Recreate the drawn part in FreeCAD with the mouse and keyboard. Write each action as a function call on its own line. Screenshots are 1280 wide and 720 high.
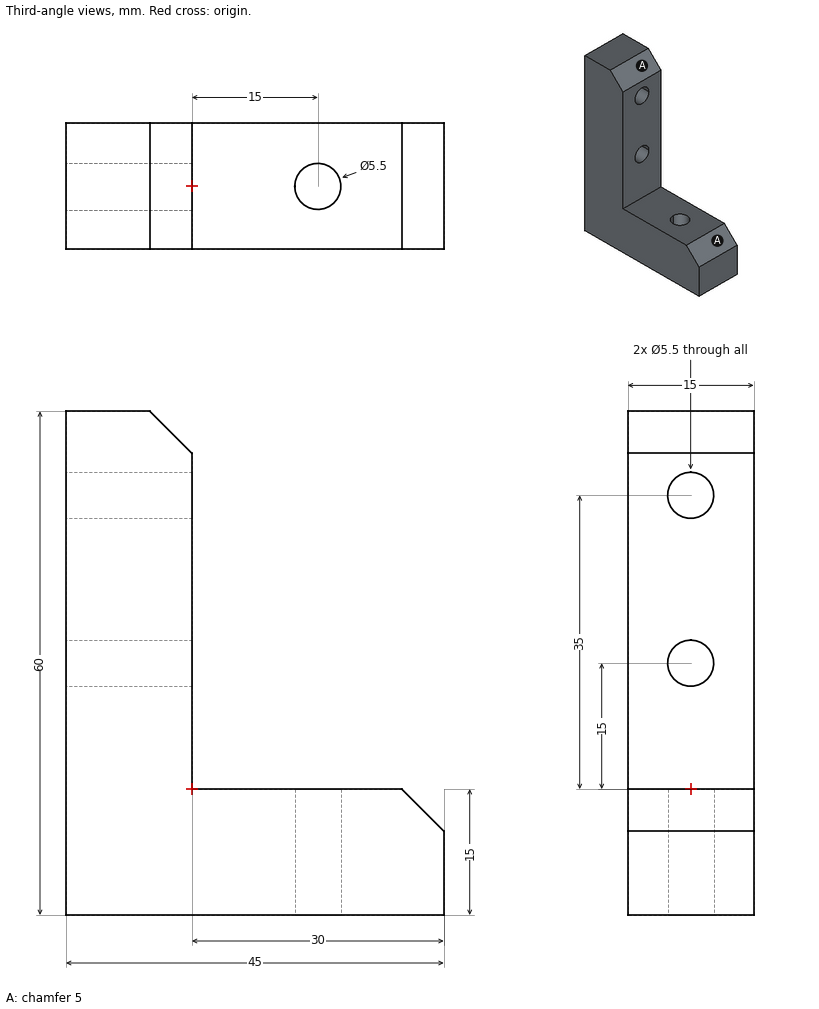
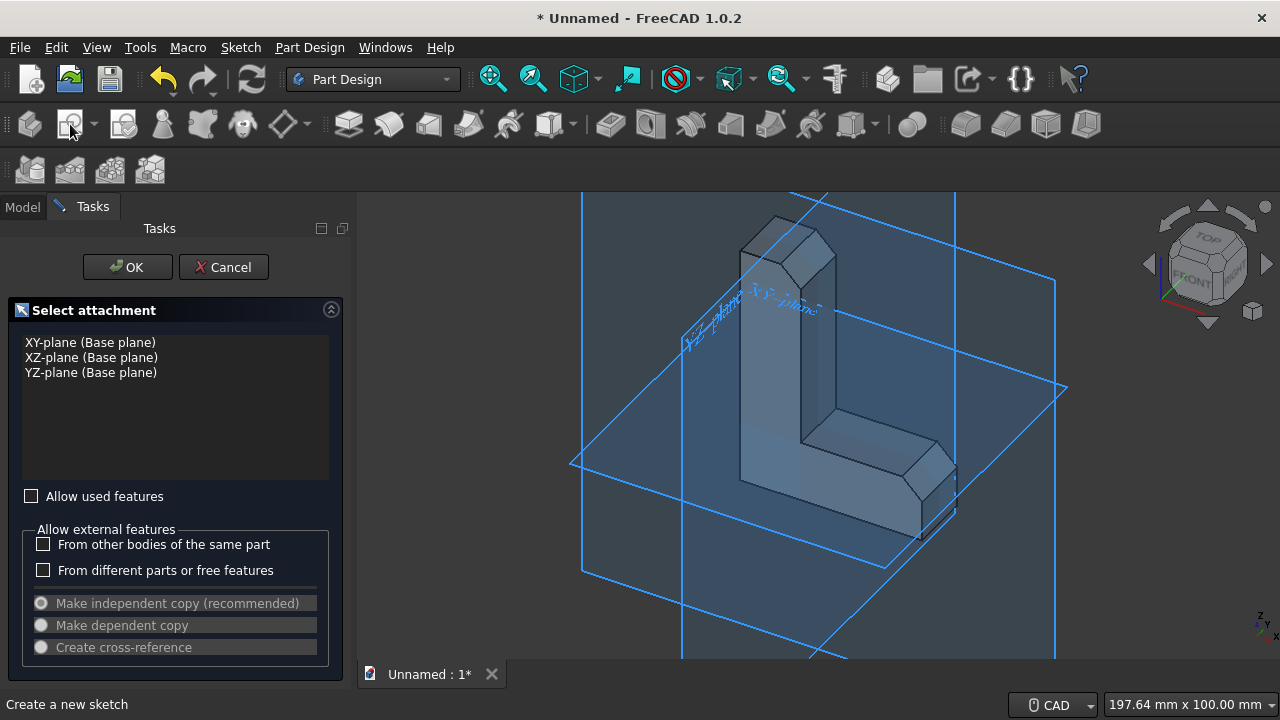
click(82, 372)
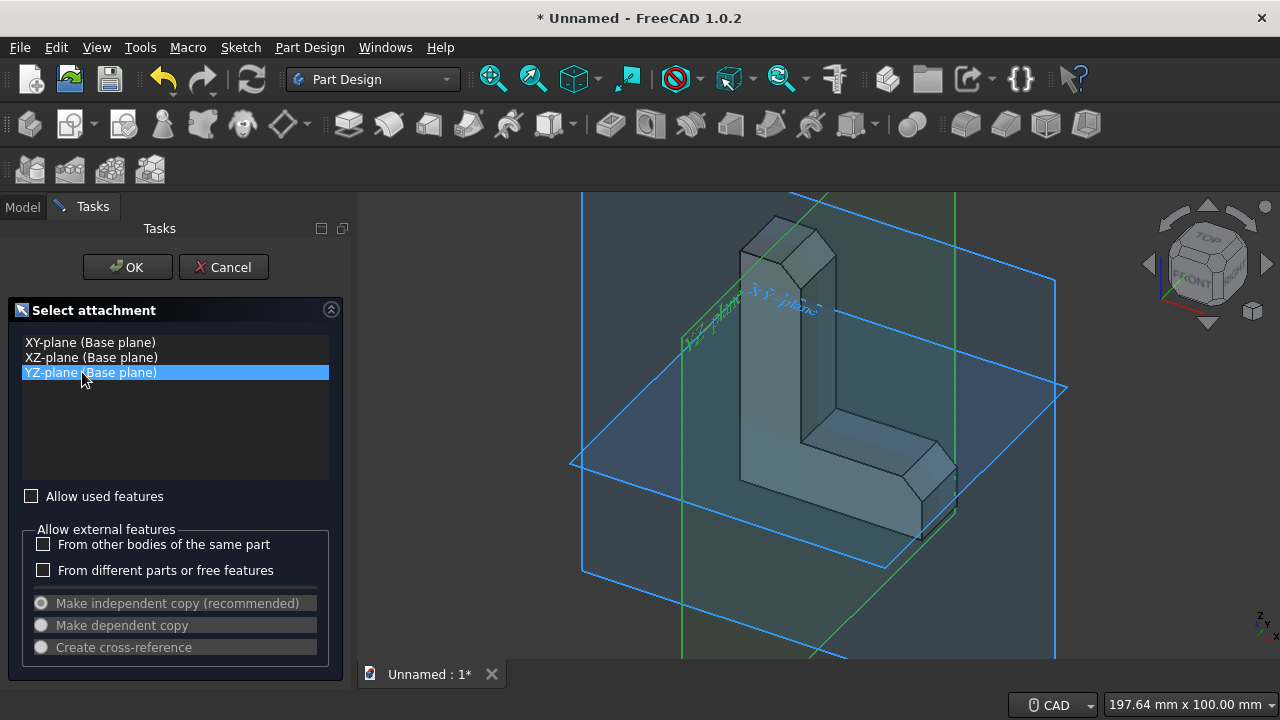
click(128, 267)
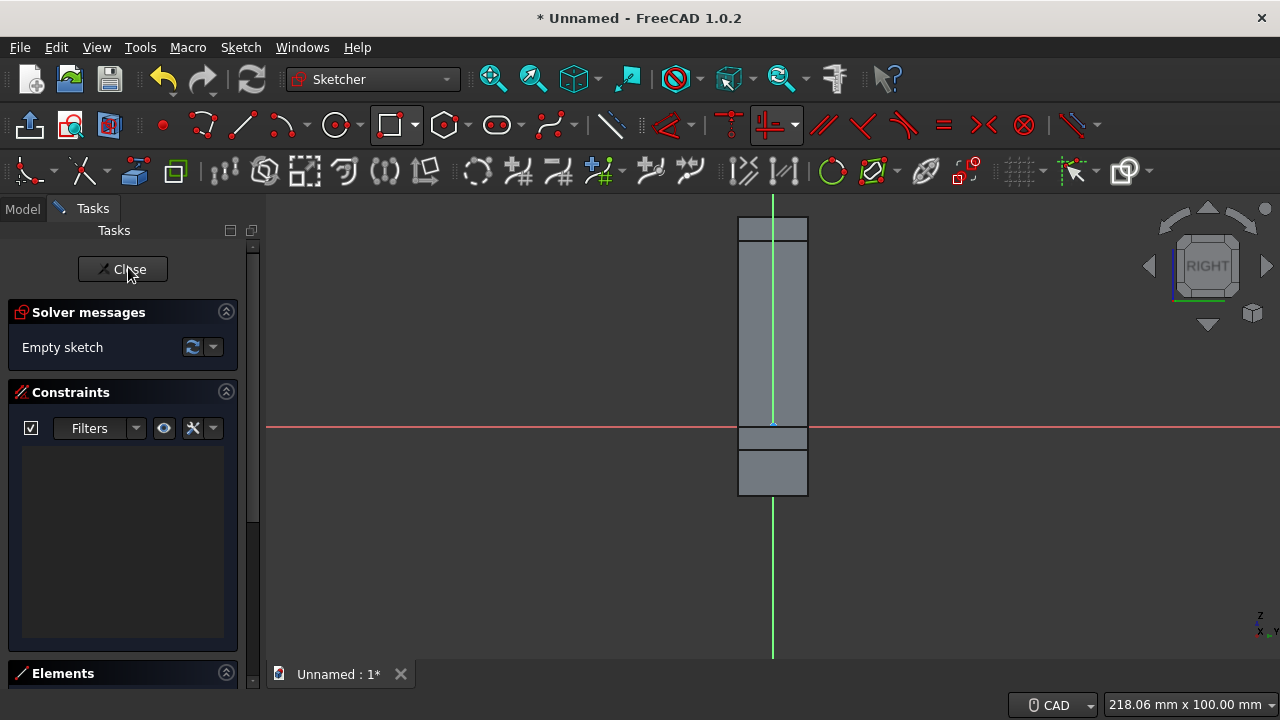
key(q)
key(s)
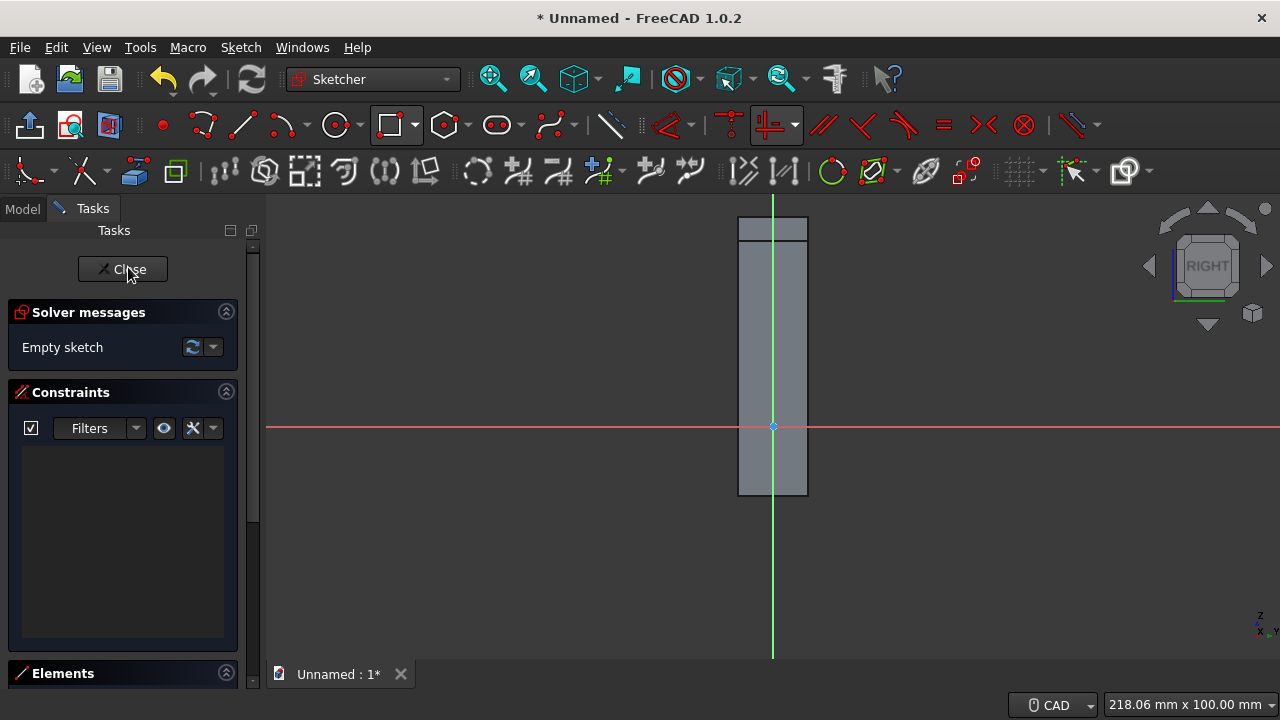
scroll(912, 222, up, 2)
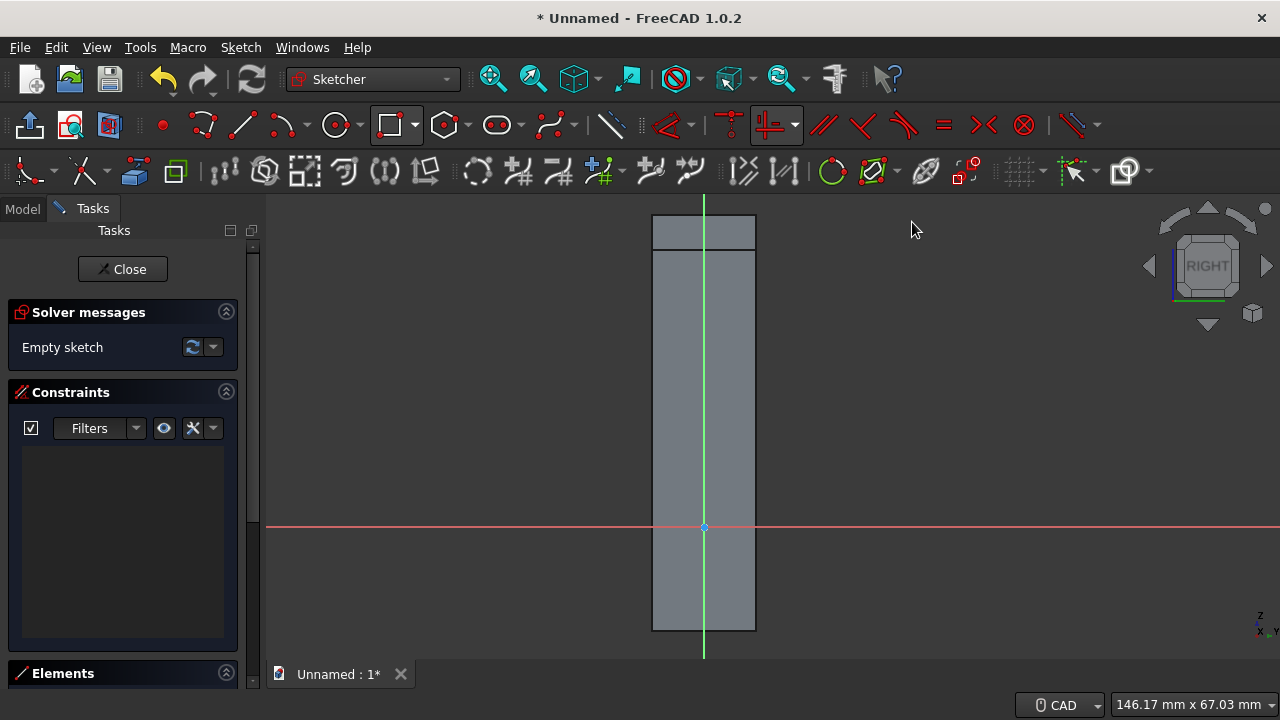
key(g)
key(c)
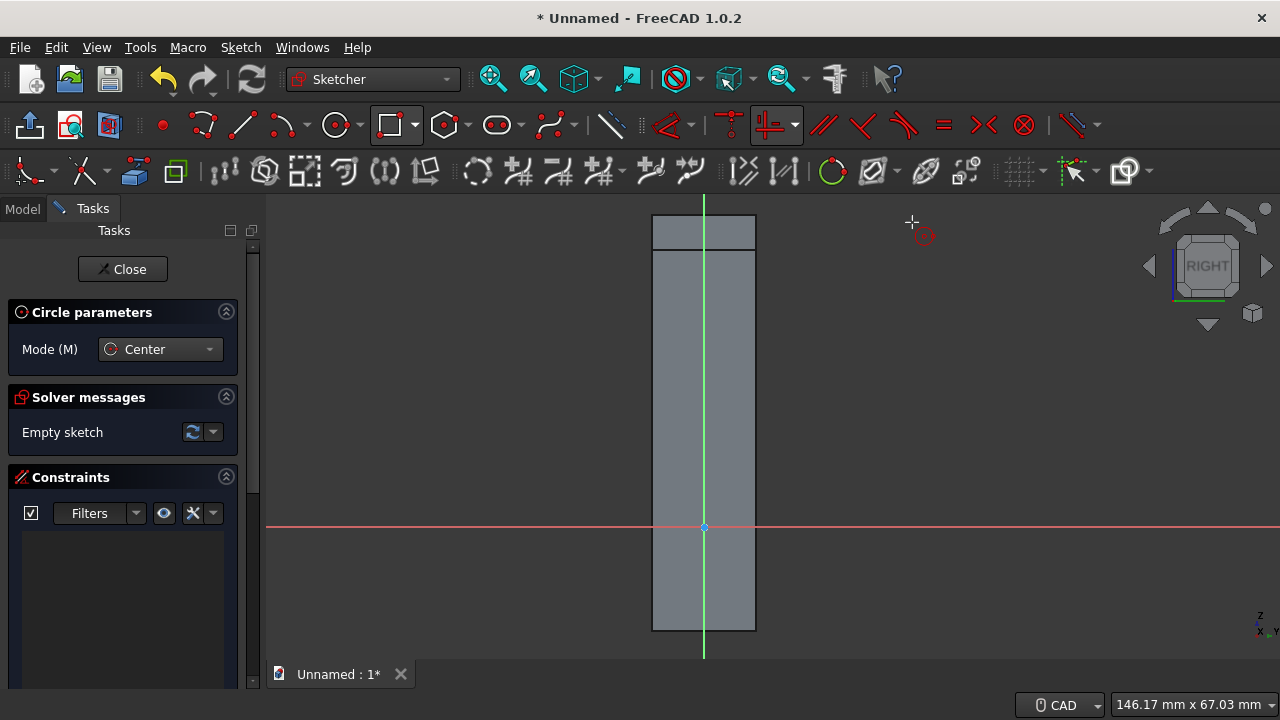
click(704, 284)
move(722, 278)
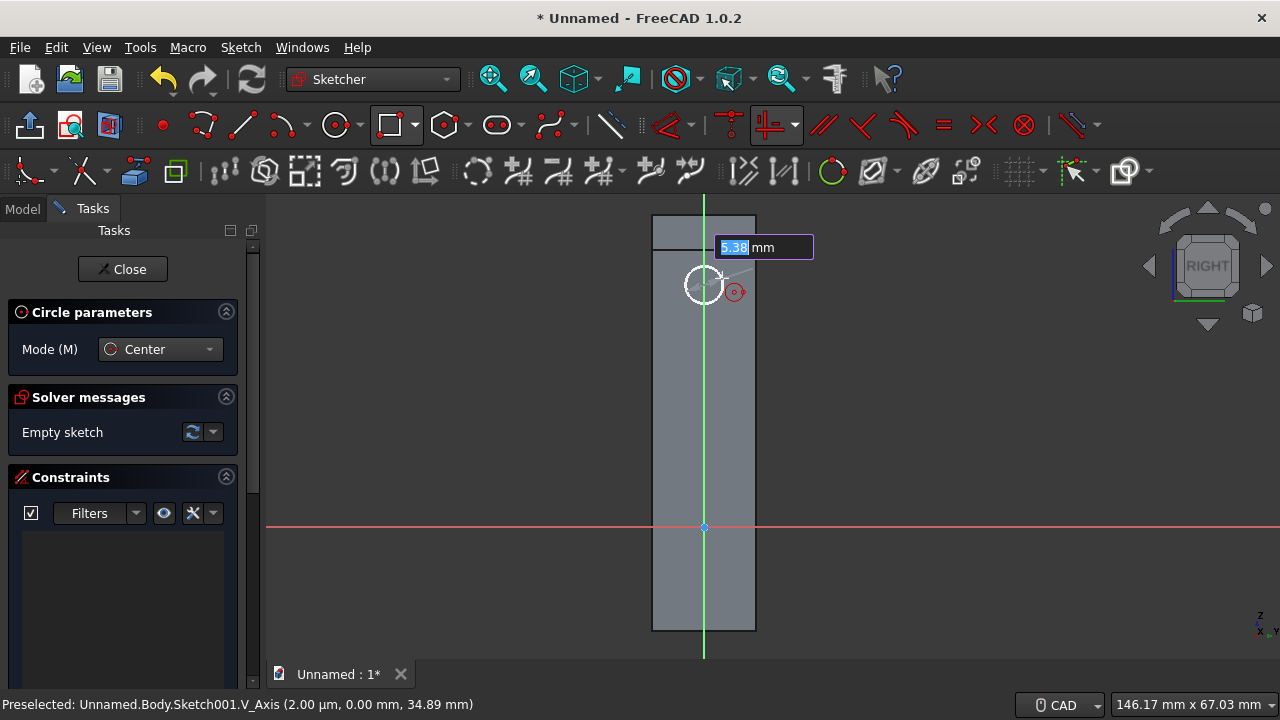
text(5.5)
key(Return)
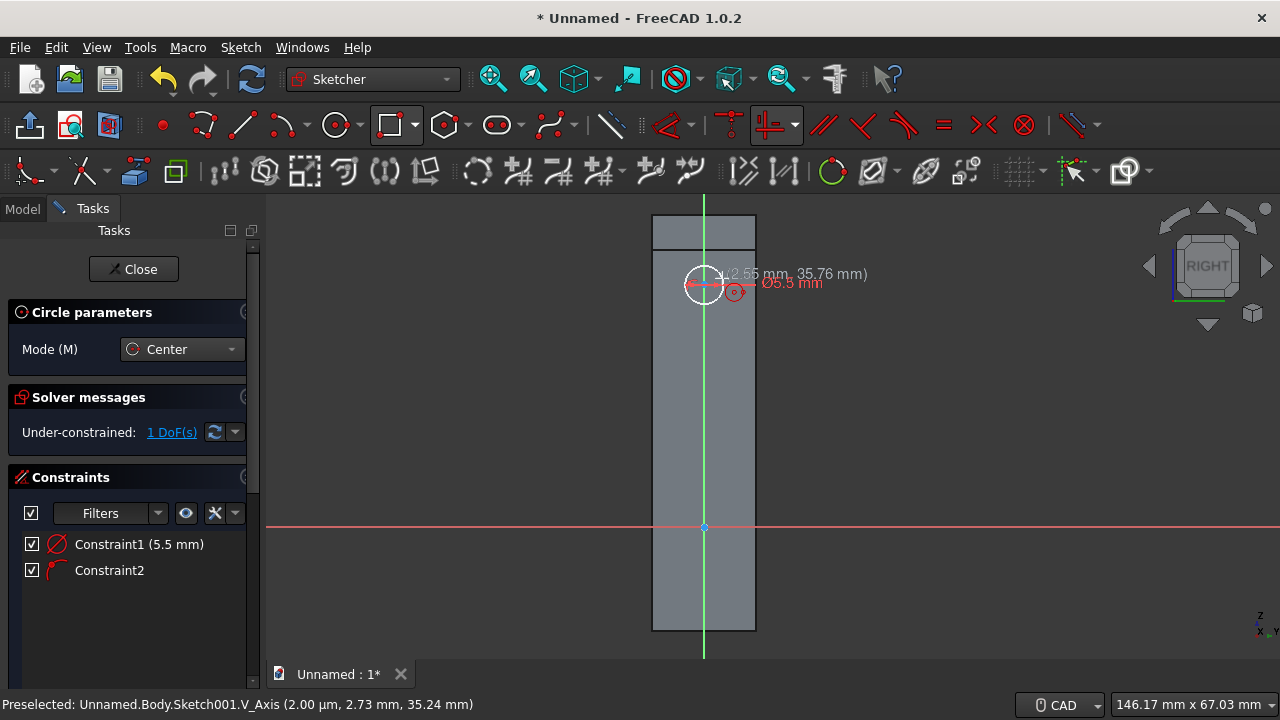
click(704, 423)
move(722, 416)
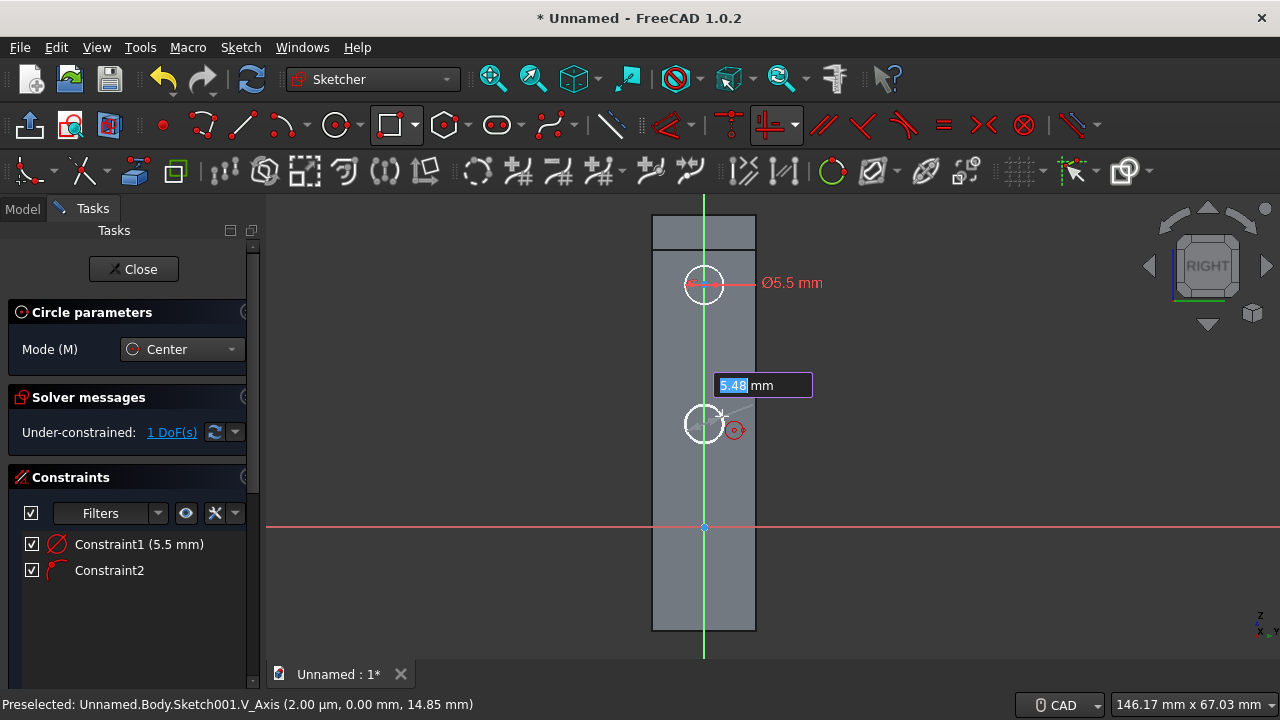
text(5.5)
key(Return)
key(Escape)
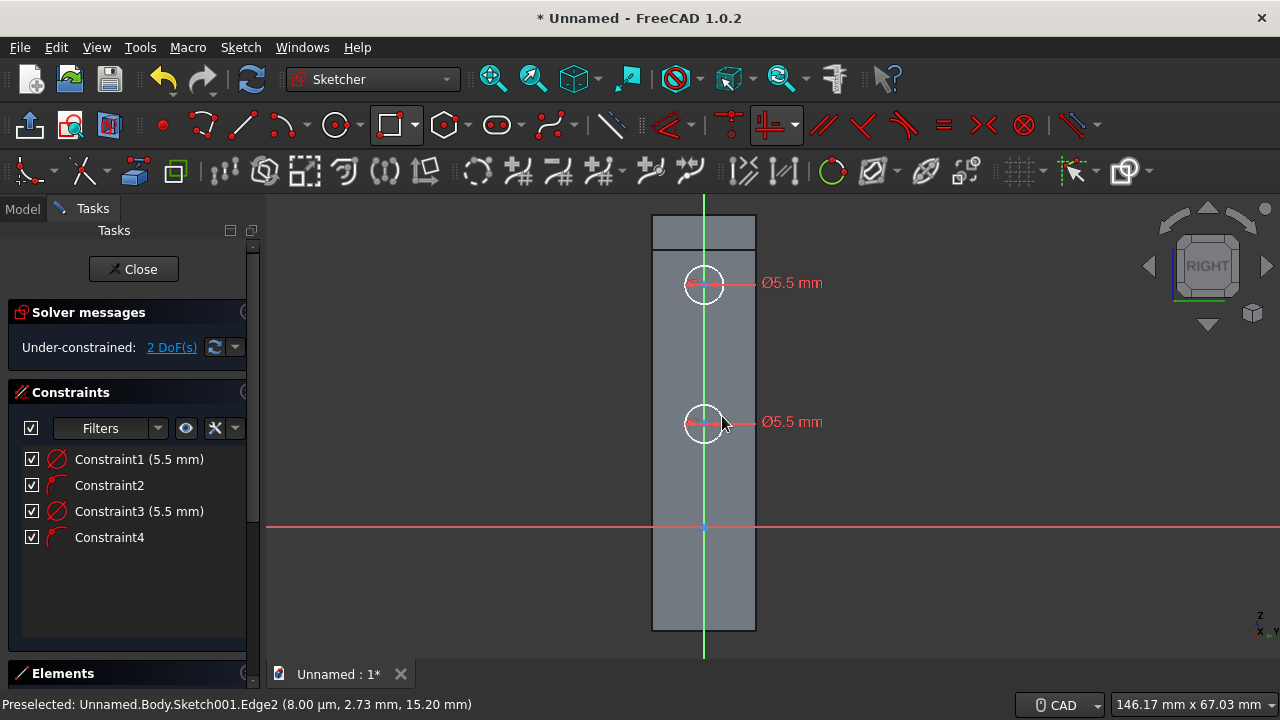
key(d)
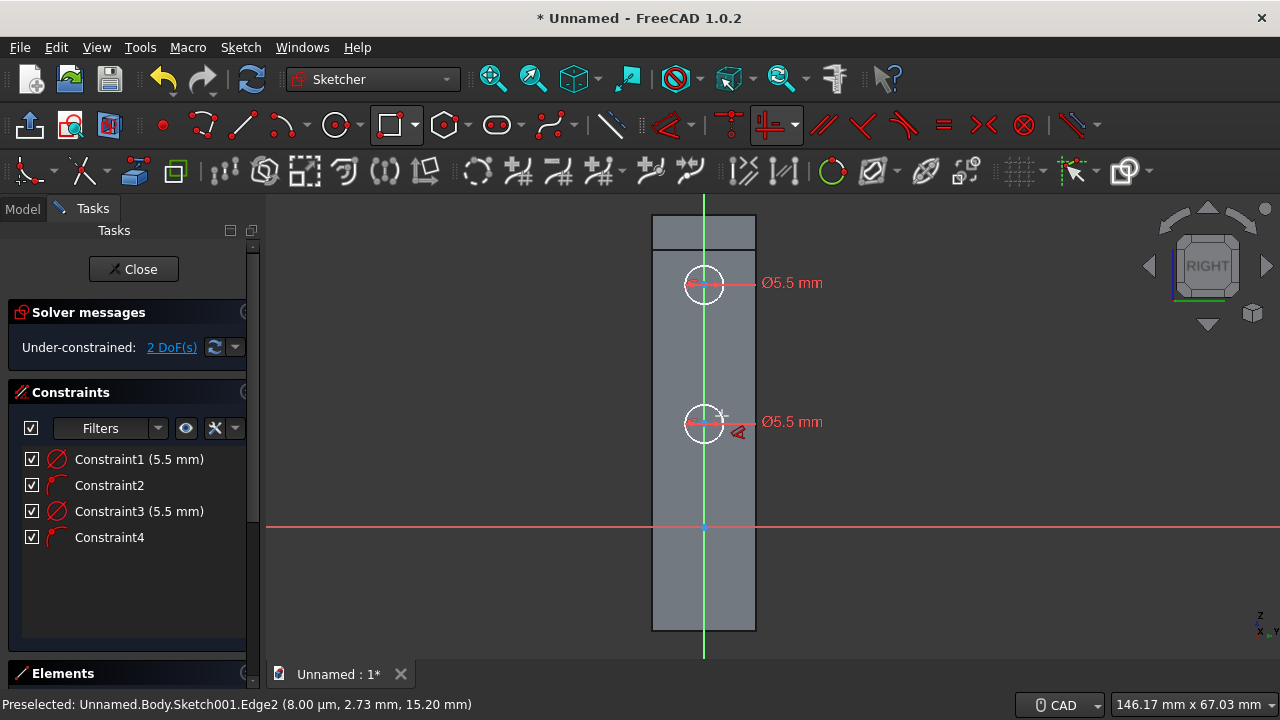
click(704, 285)
click(738, 406)